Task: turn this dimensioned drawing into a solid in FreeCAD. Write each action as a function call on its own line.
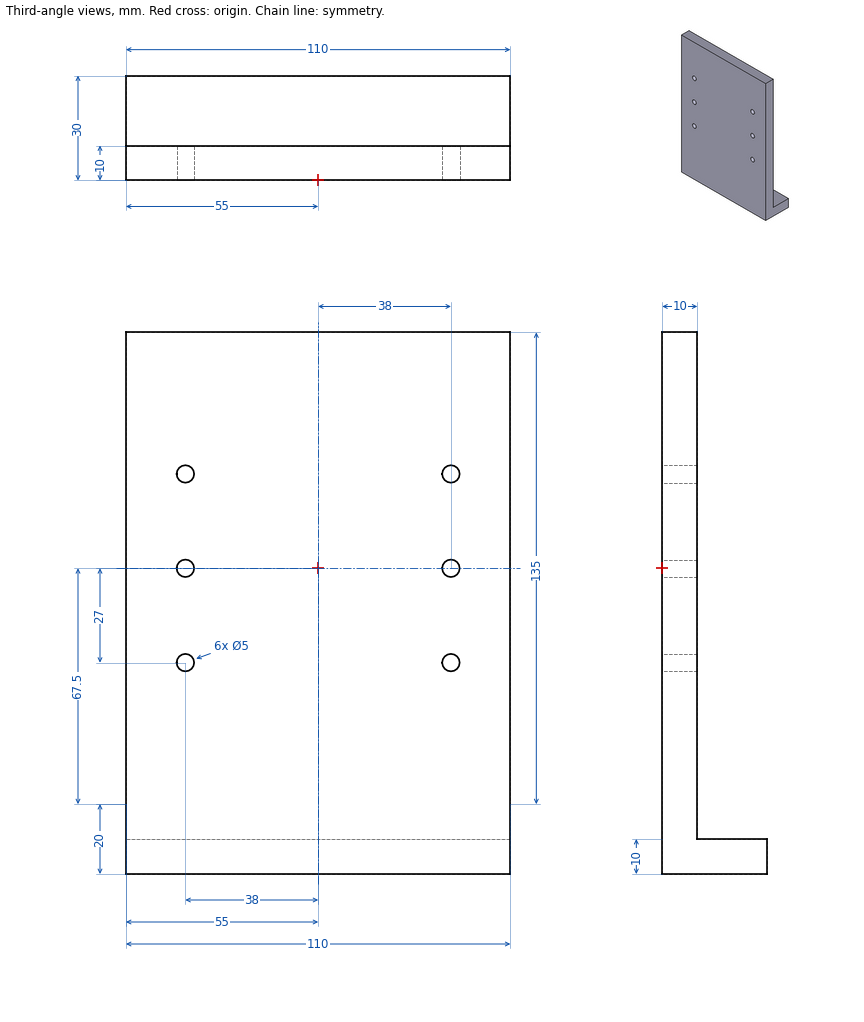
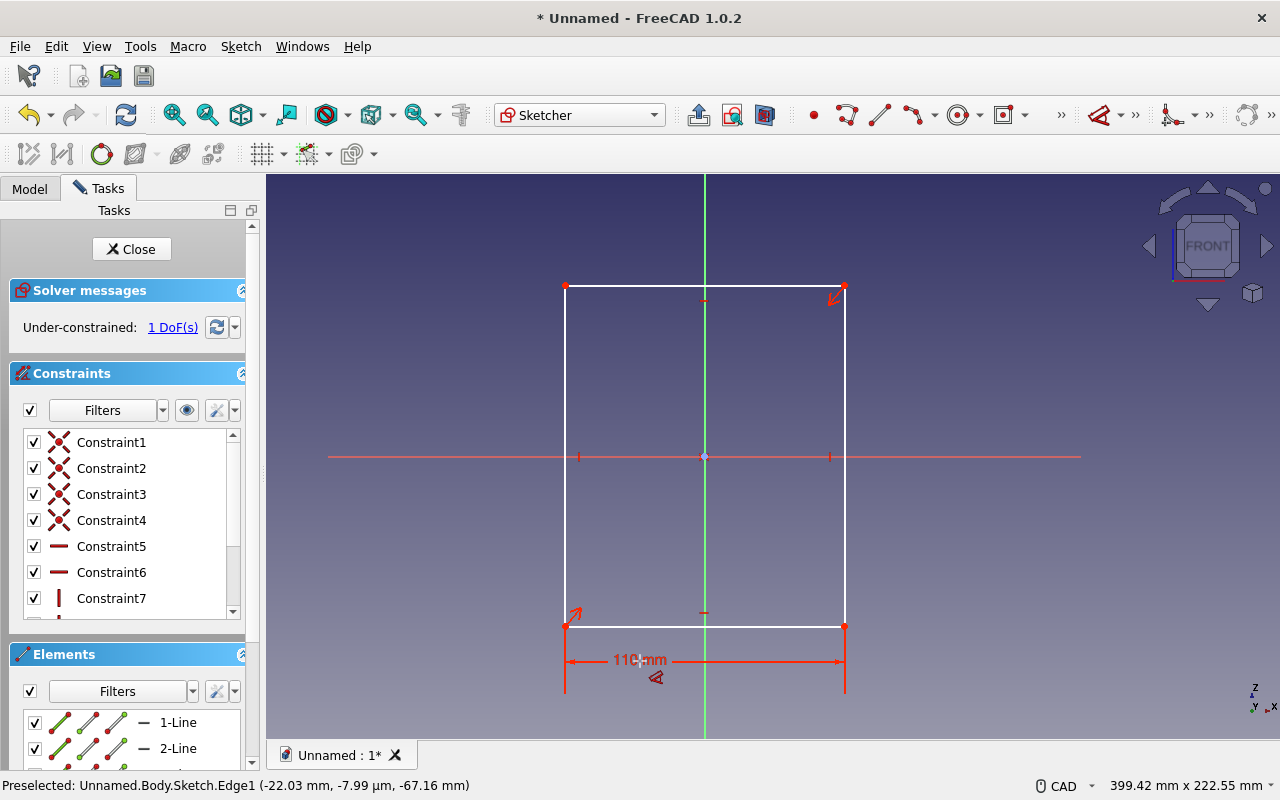
click(845, 525)
click(879, 378)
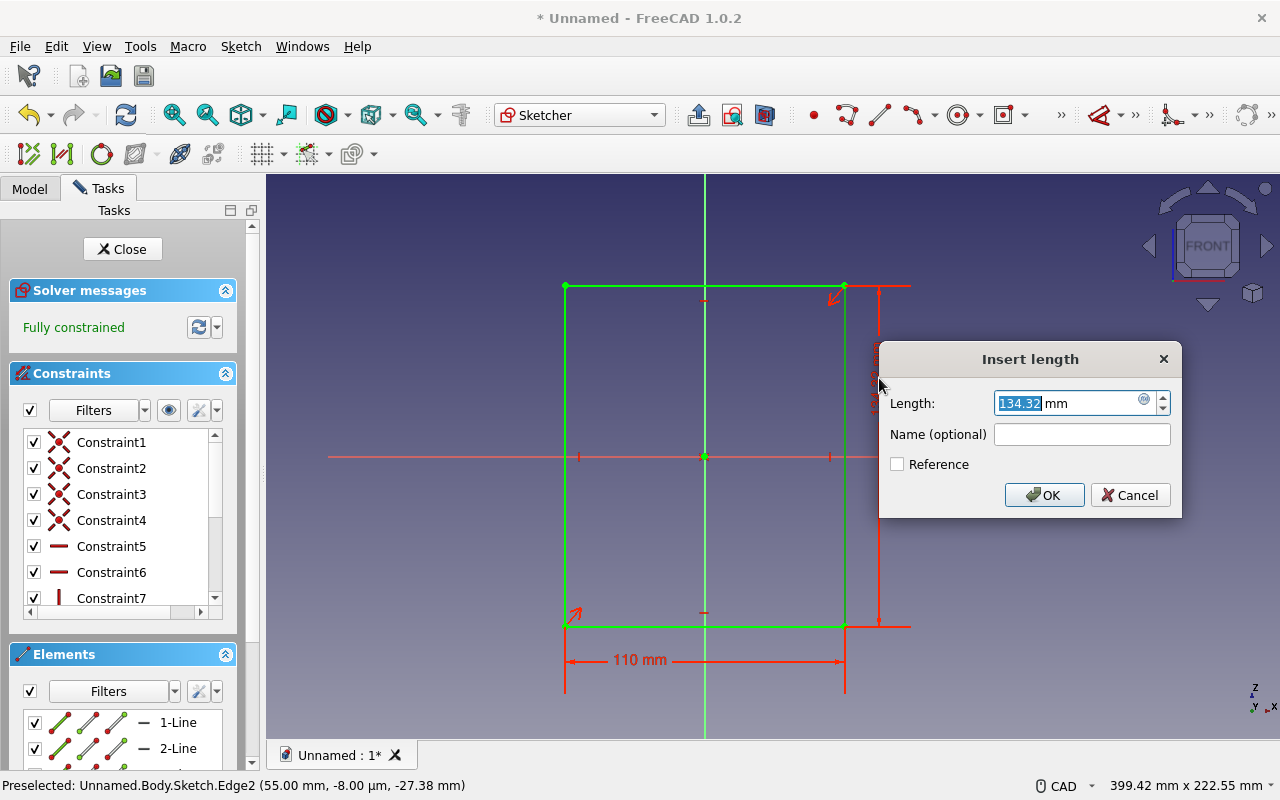
text(135)
key(Return)
key(Escape)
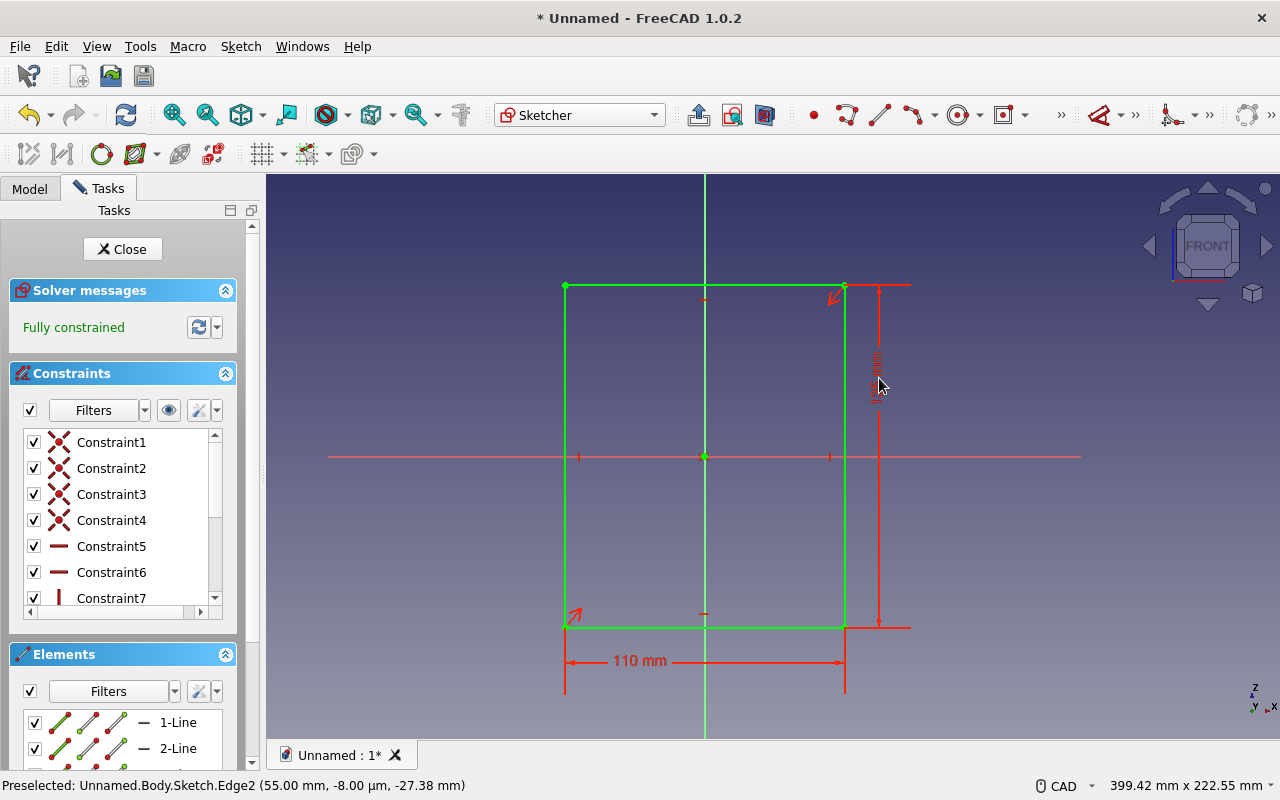
click(123, 249)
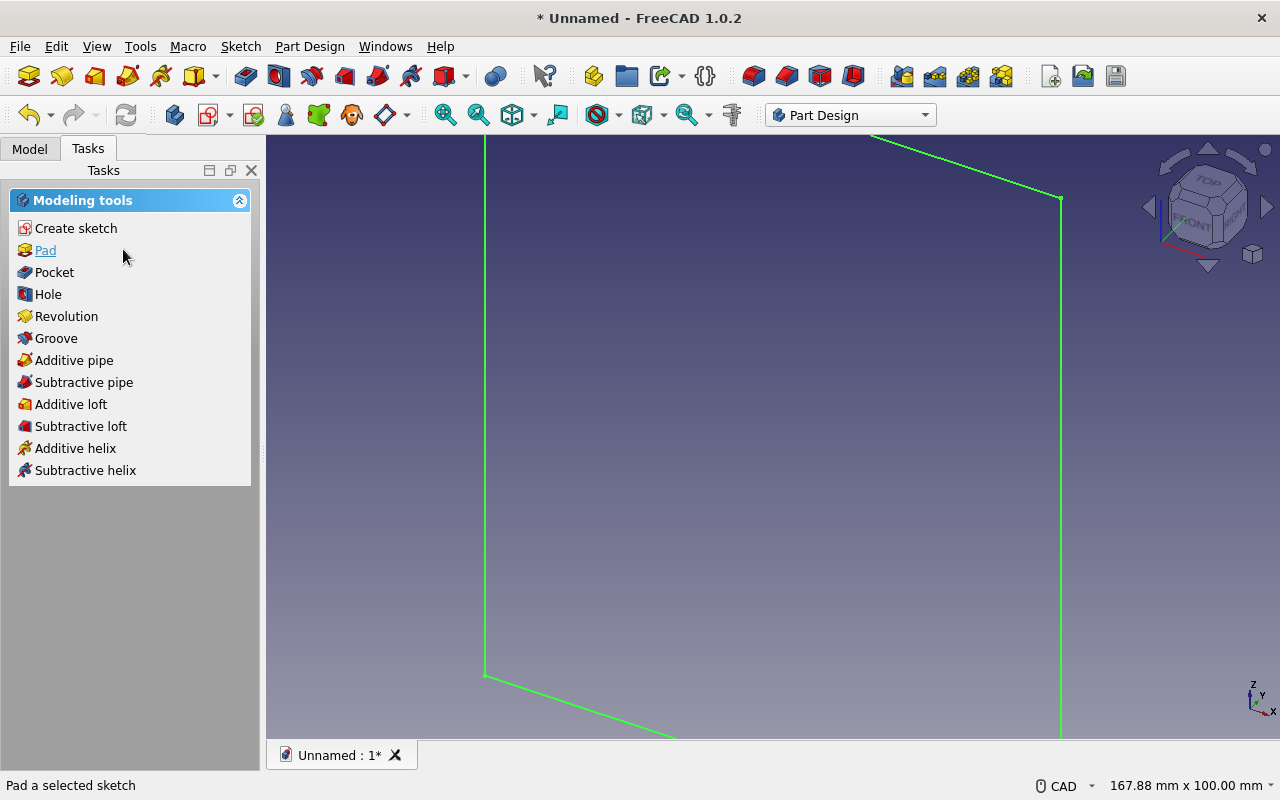
click(29, 76)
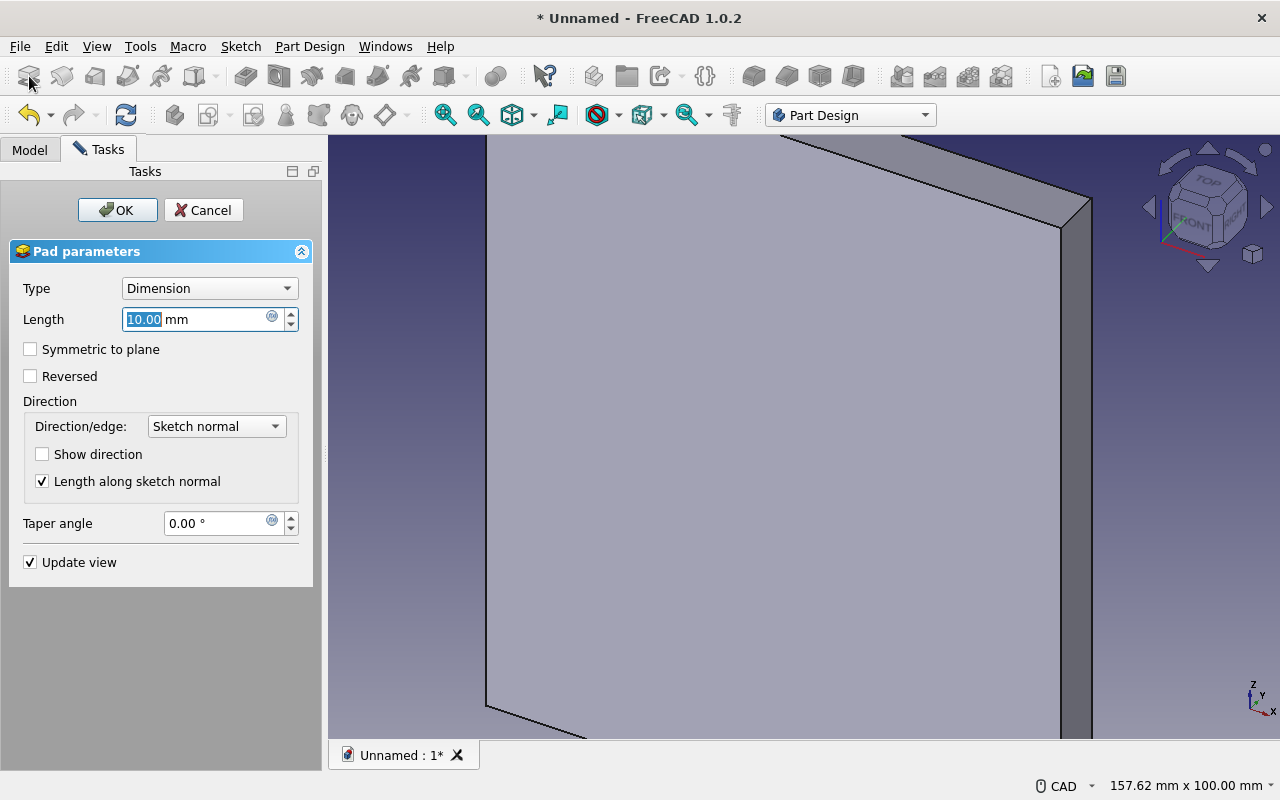
text(10)
key(Tab)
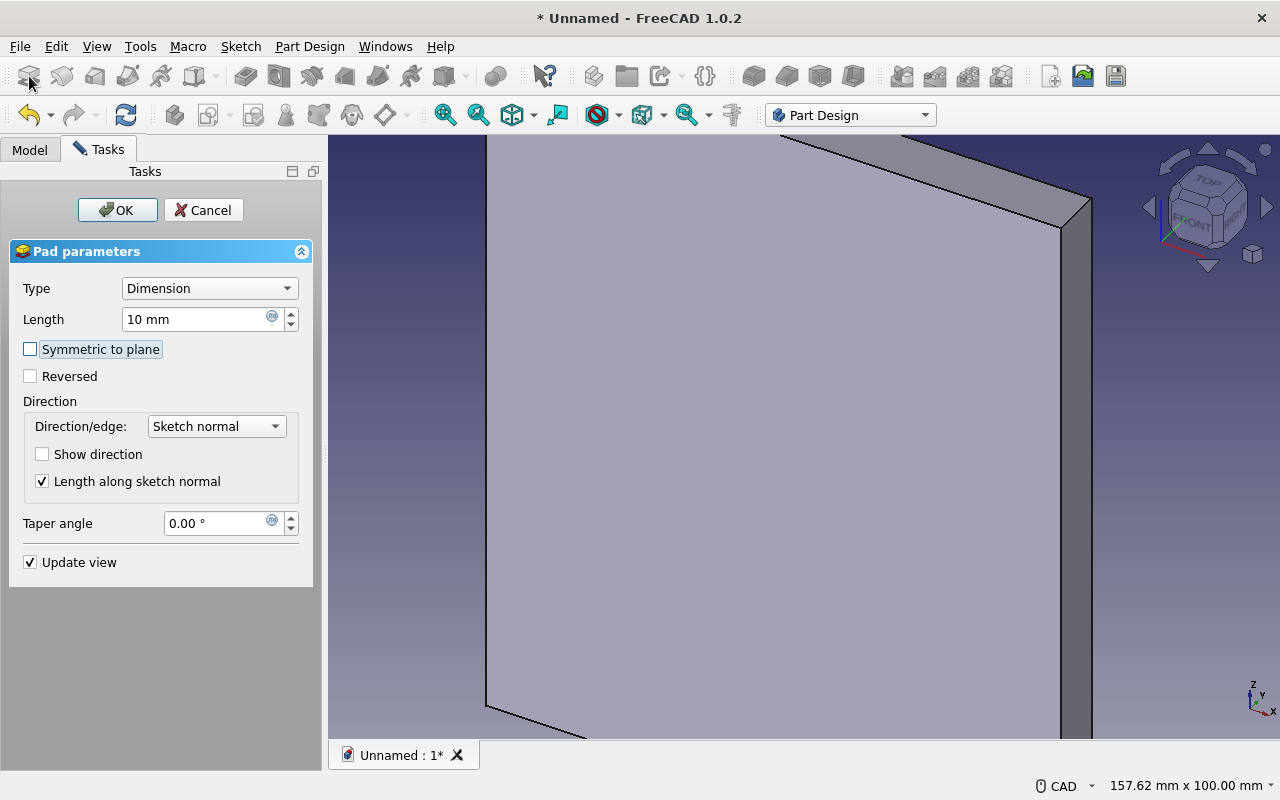
click(31, 376)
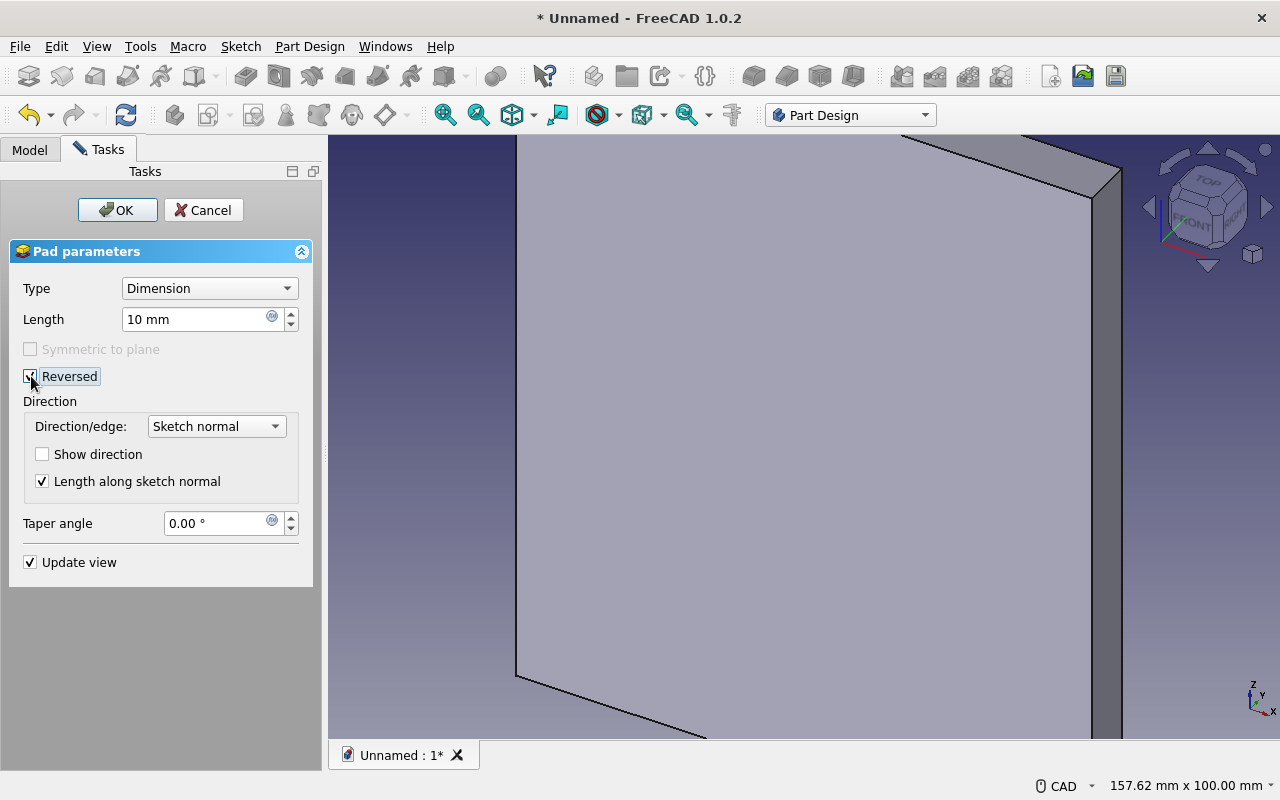
click(118, 210)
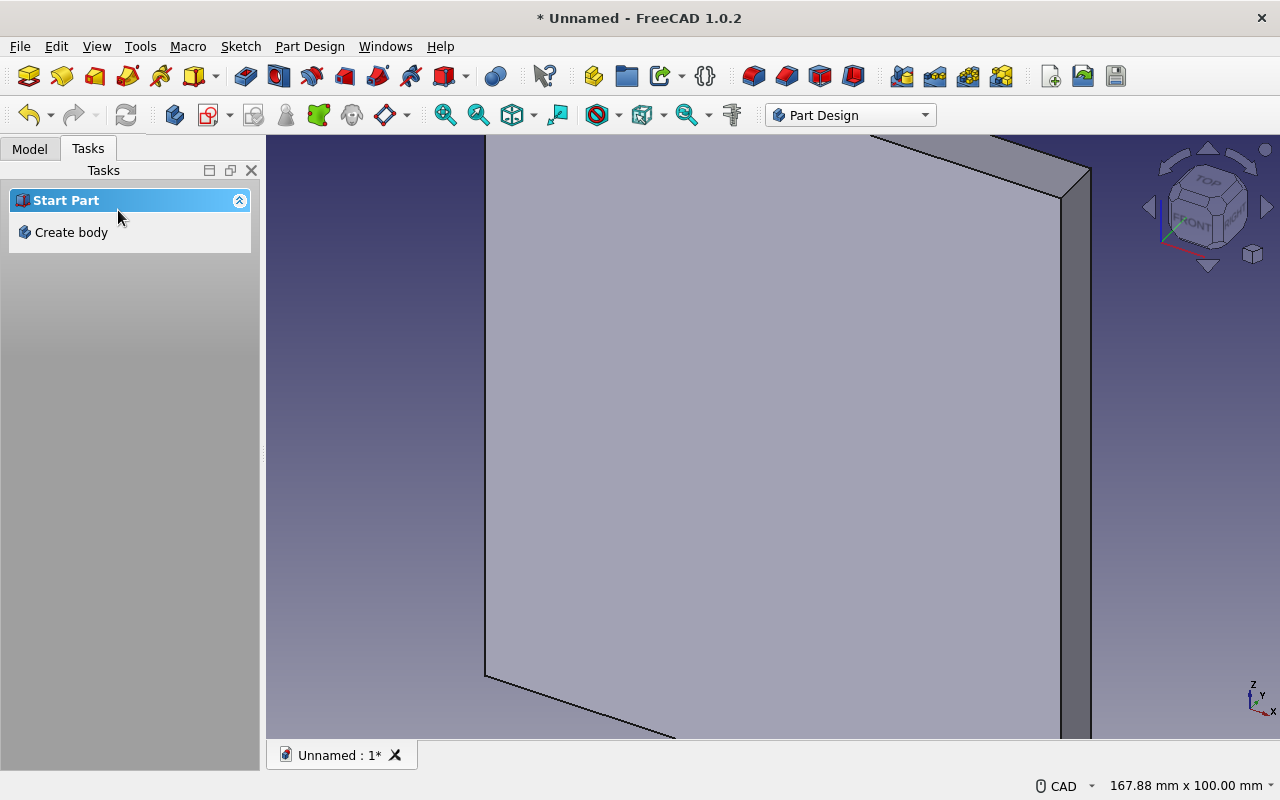
click(446, 116)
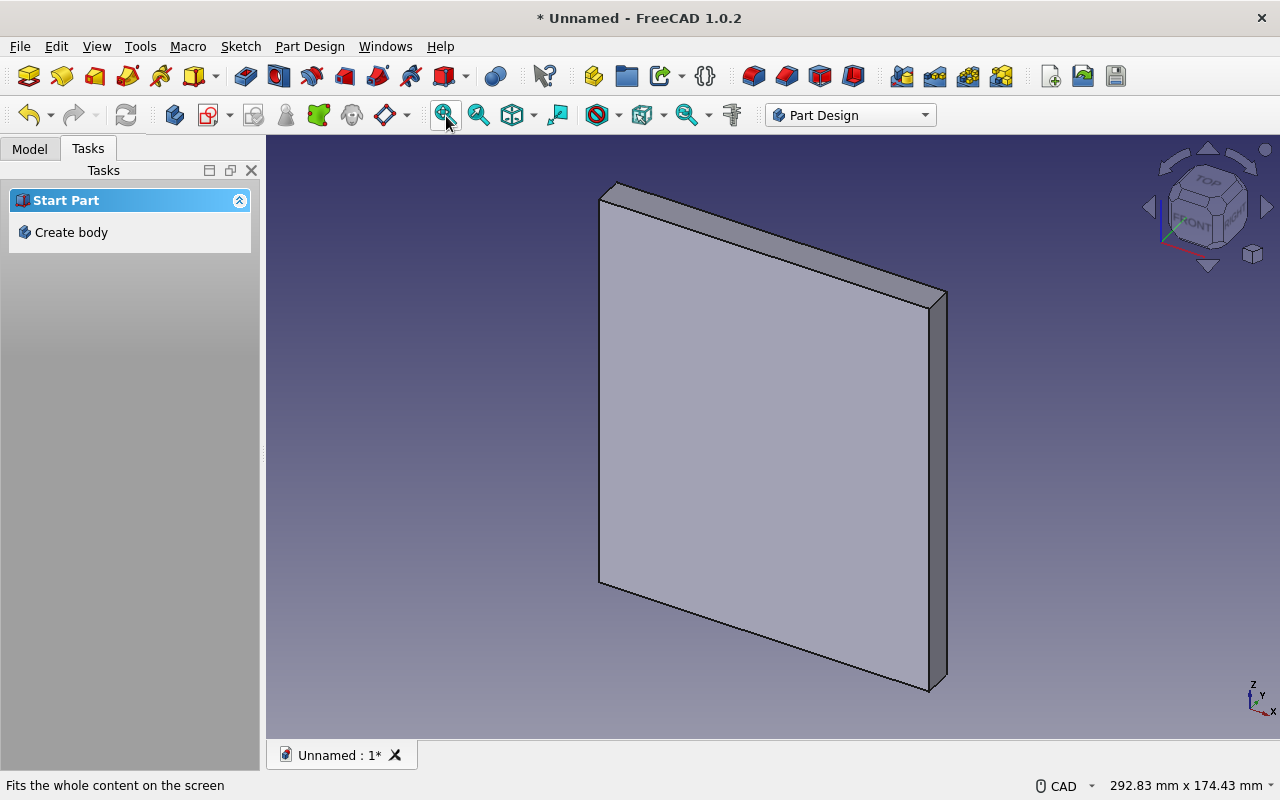
key(4)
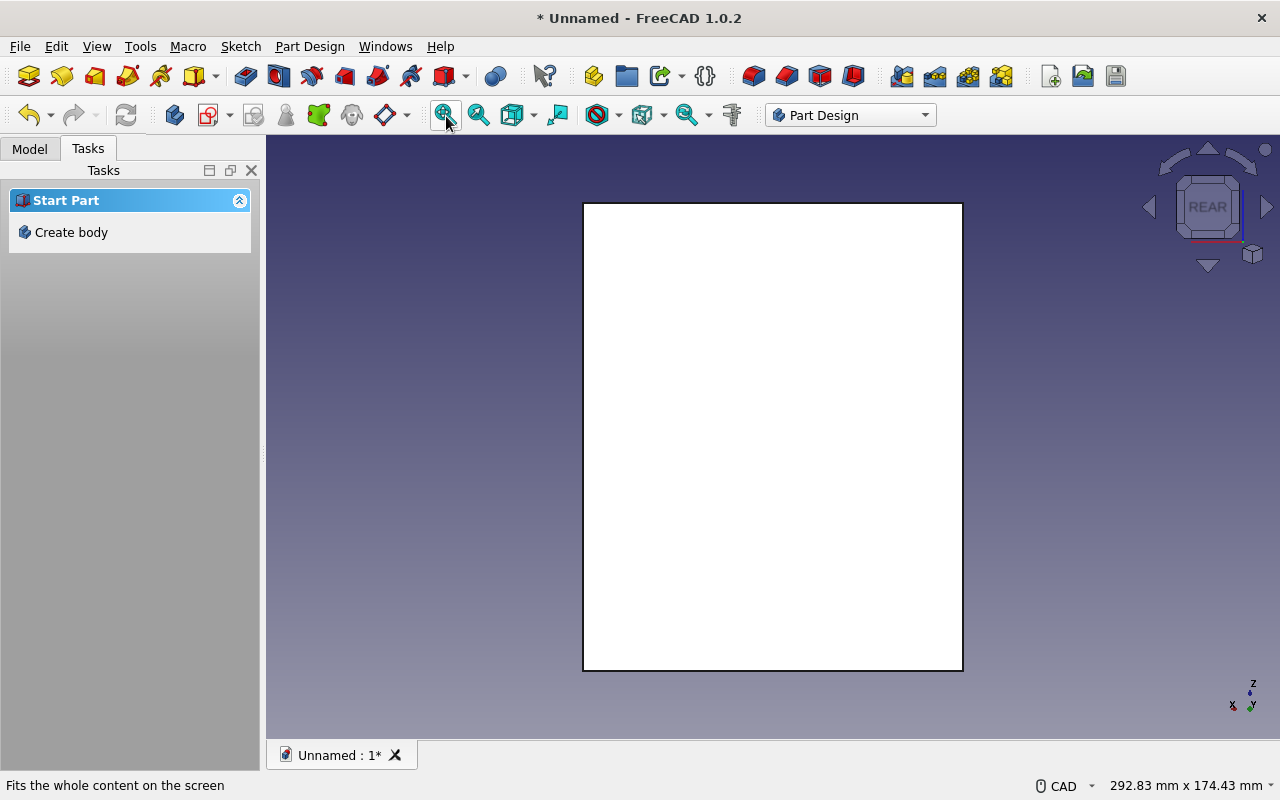
click(773, 436)